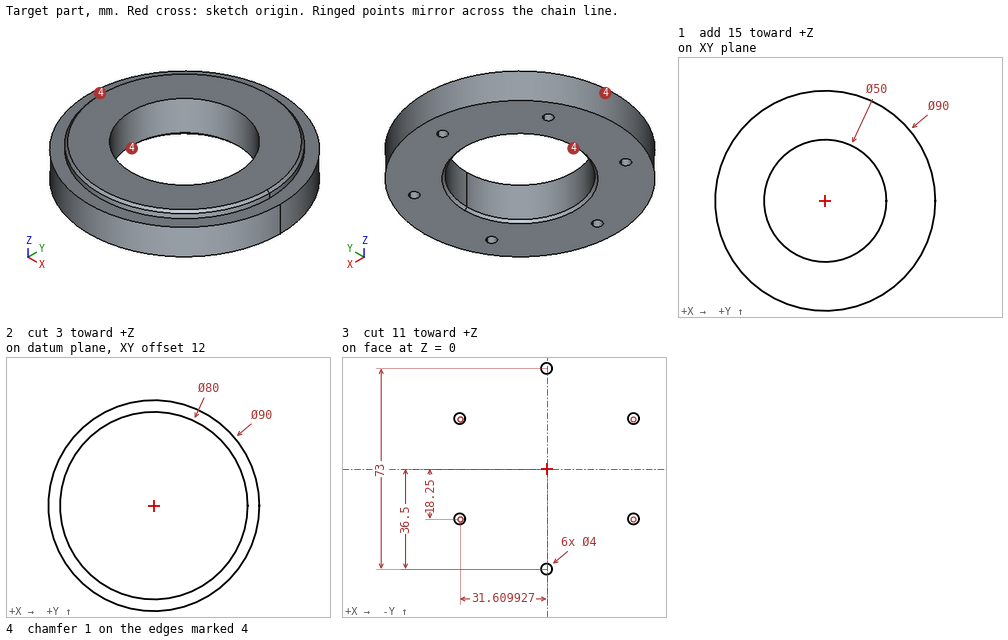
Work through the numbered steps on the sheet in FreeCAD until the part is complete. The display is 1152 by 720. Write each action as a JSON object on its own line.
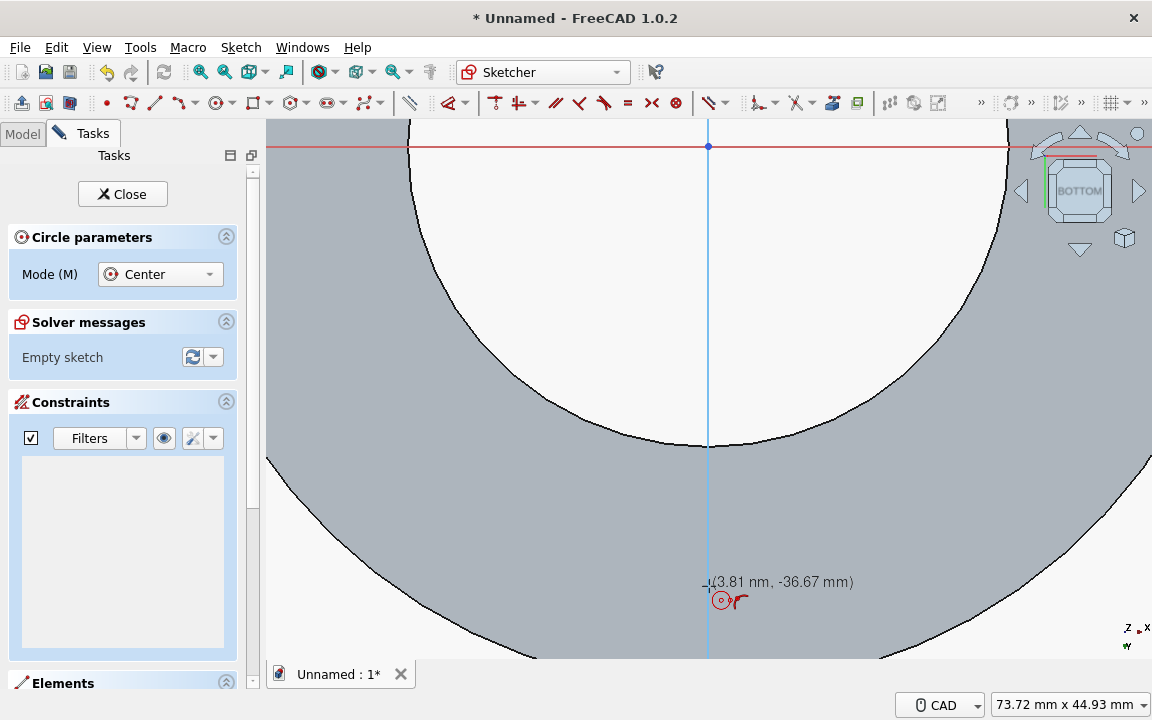
{"action": "left_click", "coordinate": [708, 585]}
{"action": "left_click", "coordinate": [725, 568]}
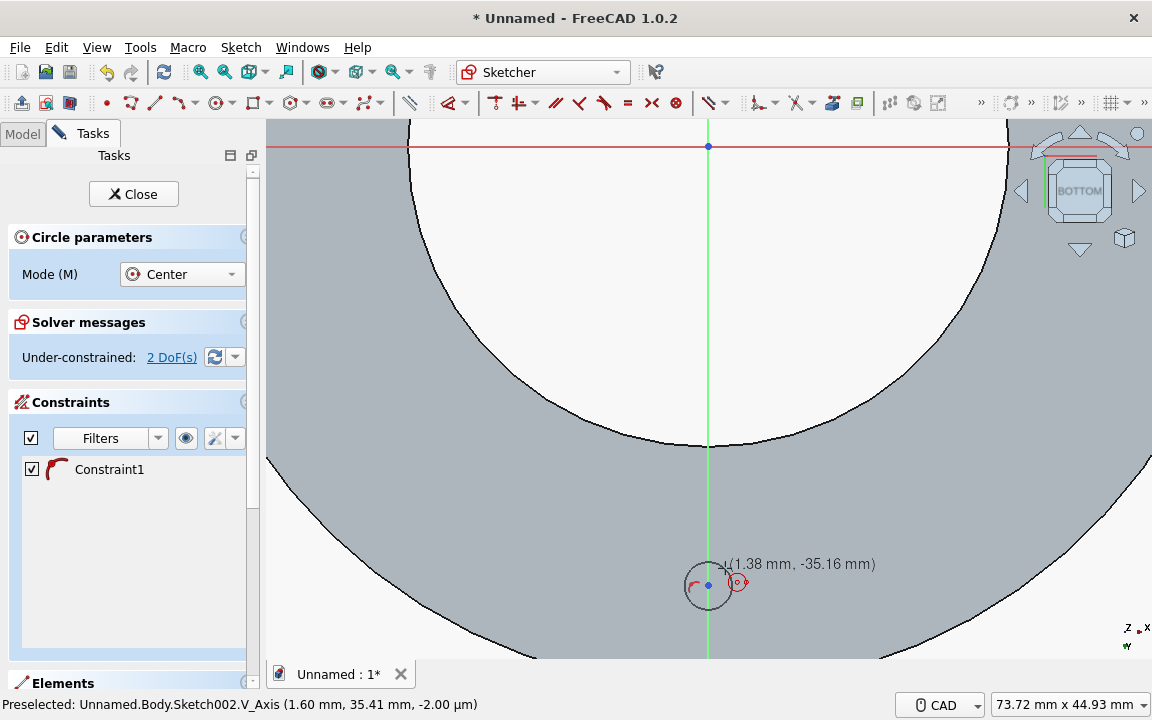
{"action": "left_click", "coordinate": [329, 366]}
{"action": "left_click", "coordinate": [345, 349]}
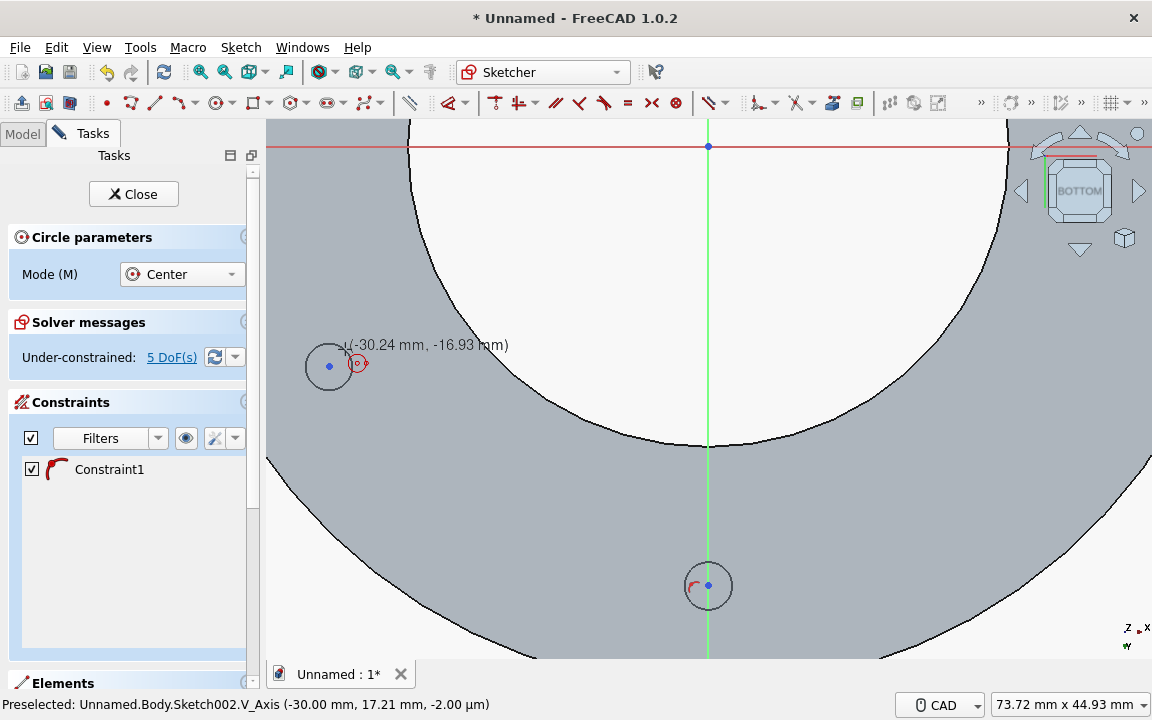
{"action": "scroll", "coordinate": [601, 530], "scroll_direction": "down", "scroll_amount": 5}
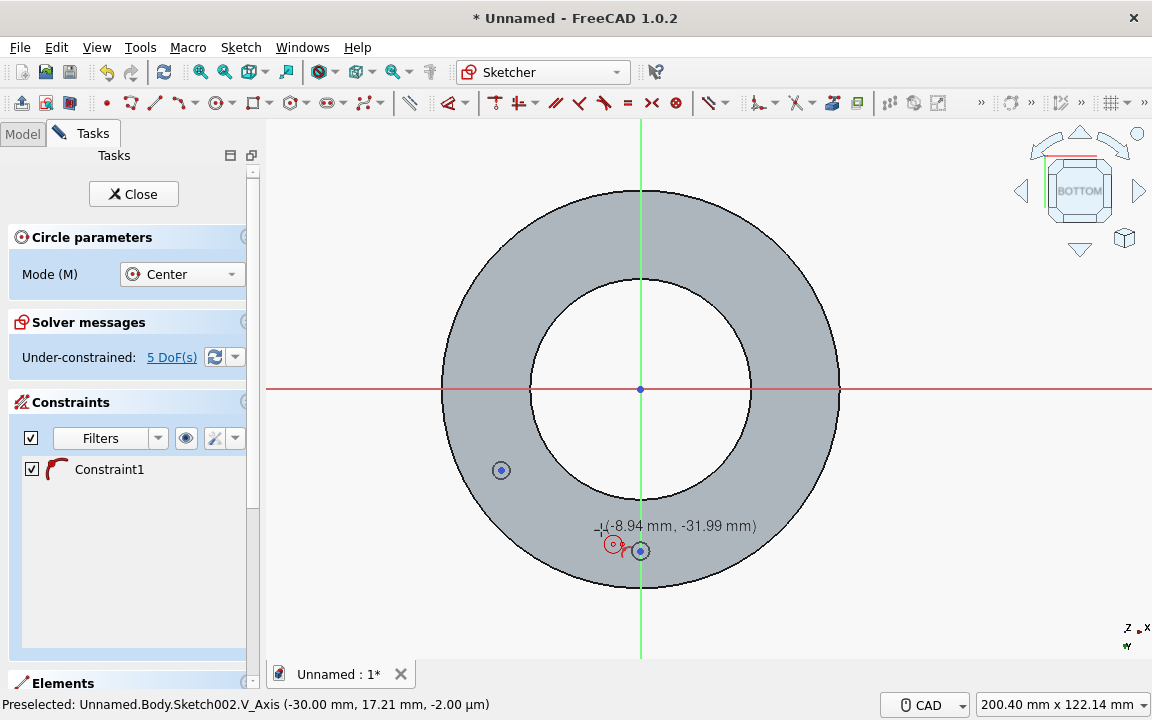
{"action": "scroll", "coordinate": [501, 309], "scroll_direction": "up", "scroll_amount": 5}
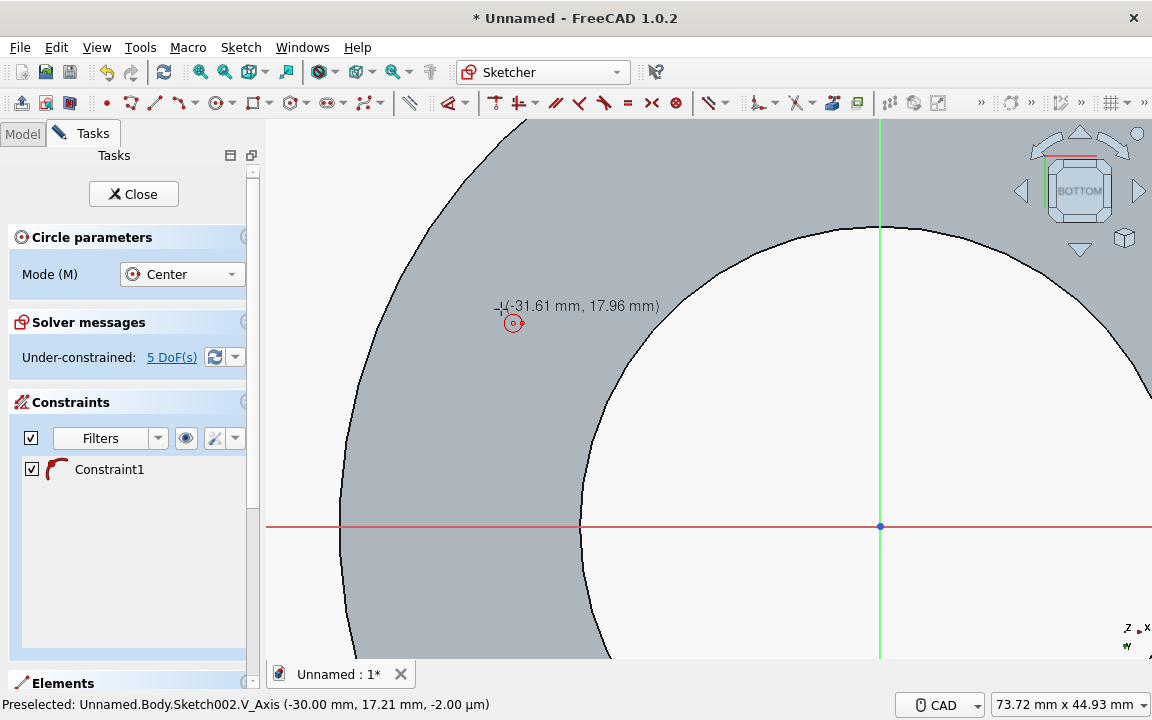
{"action": "left_click", "coordinate": [501, 308]}
{"action": "left_click", "coordinate": [518, 291]}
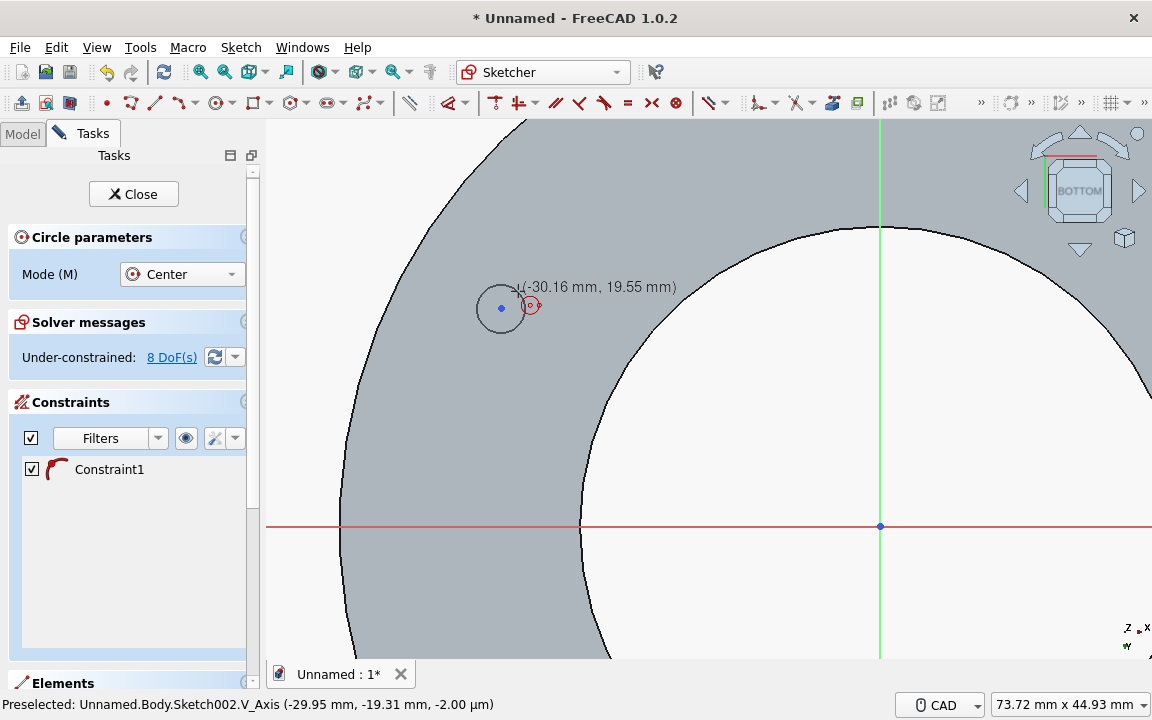
{"action": "scroll", "coordinate": [501, 309], "scroll_direction": "down", "scroll_amount": 5}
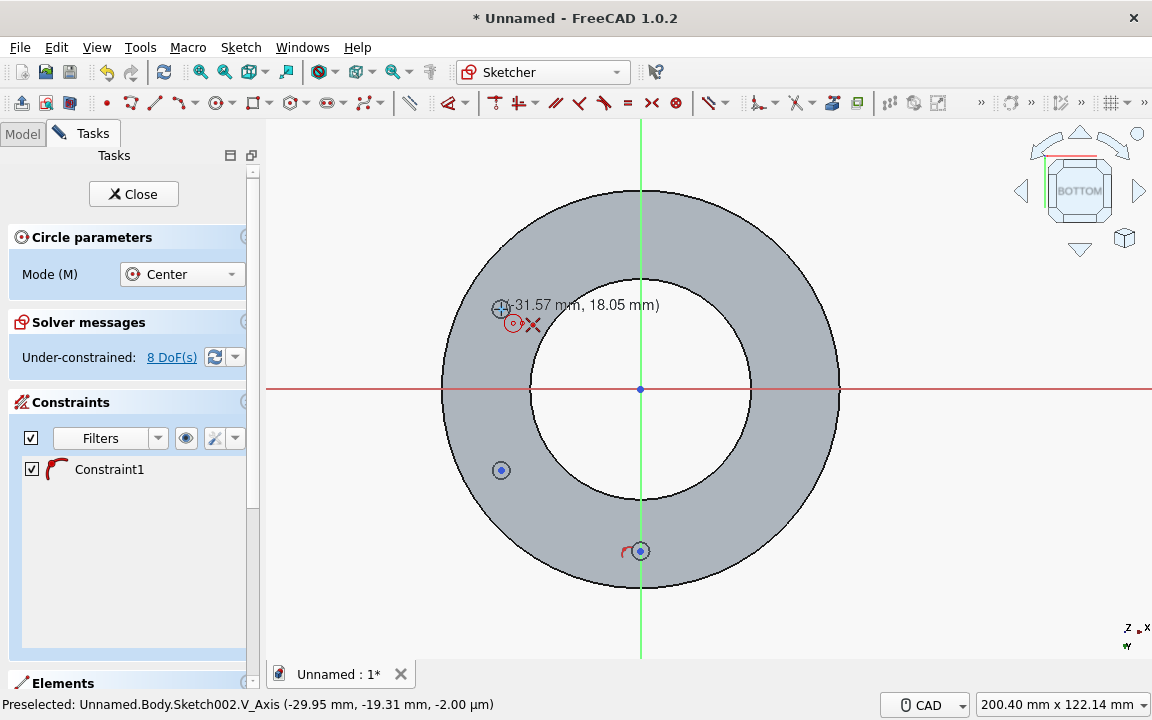
{"action": "scroll", "coordinate": [641, 228], "scroll_direction": "up", "scroll_amount": 5}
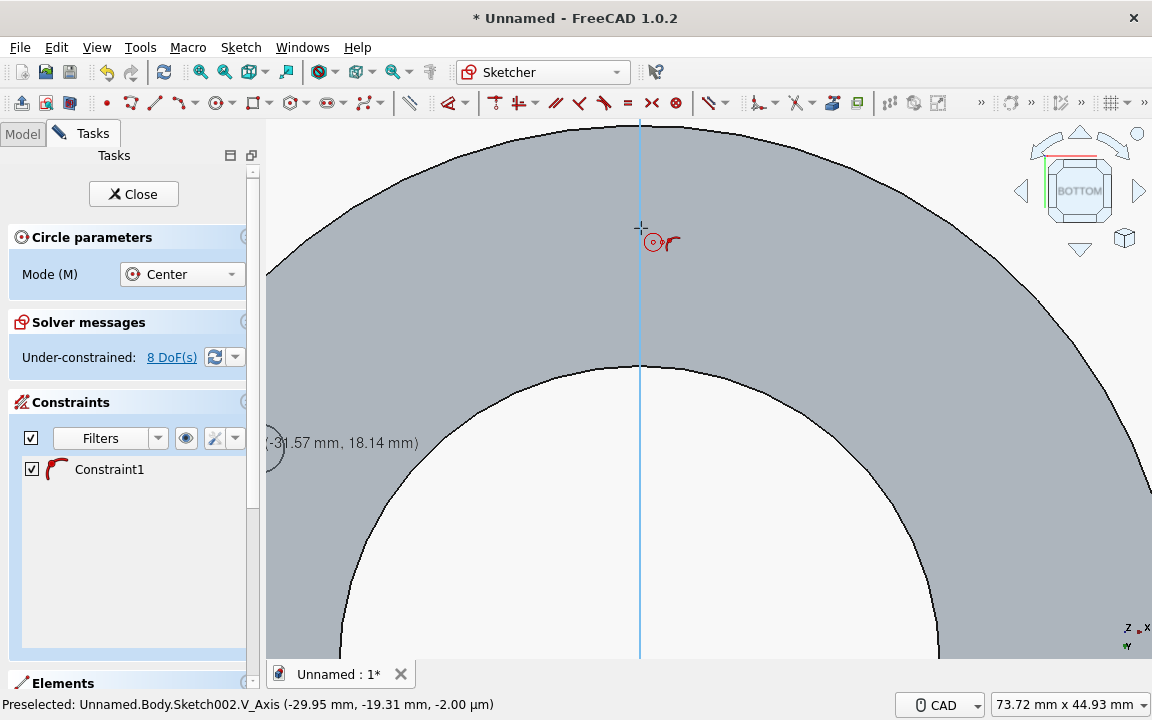
{"action": "left_click", "coordinate": [640, 228]}
{"action": "left_click", "coordinate": [657, 211]}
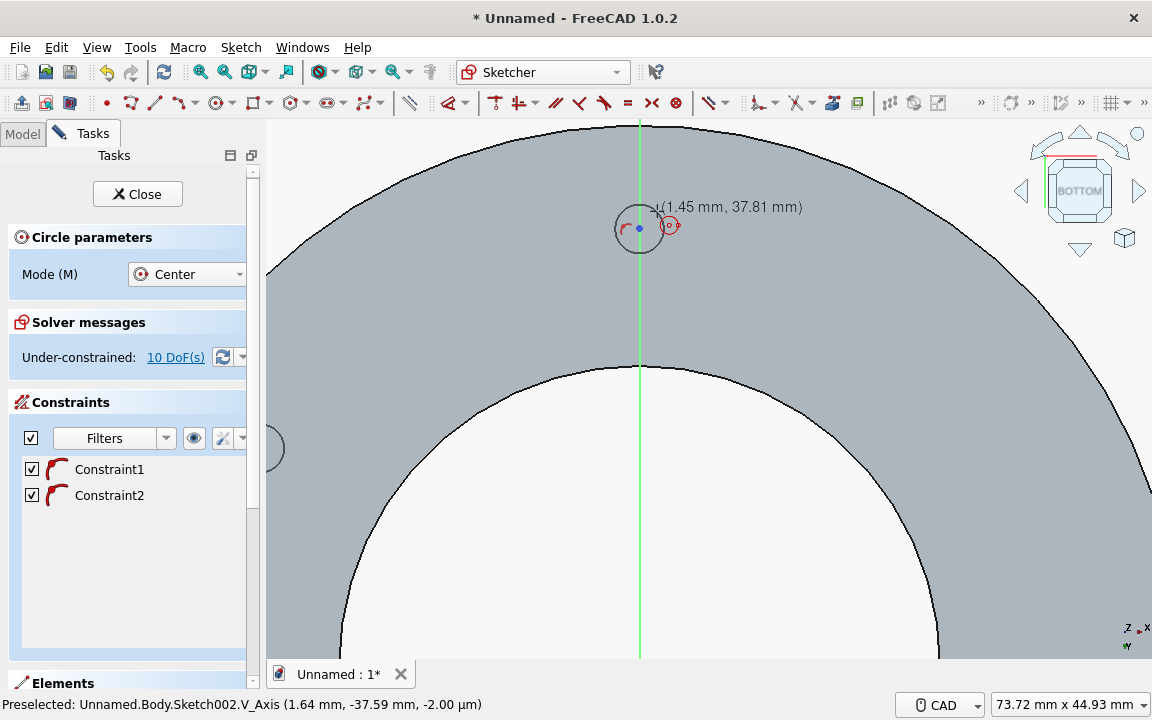
{"action": "scroll", "coordinate": [641, 228], "scroll_direction": "down", "scroll_amount": 5}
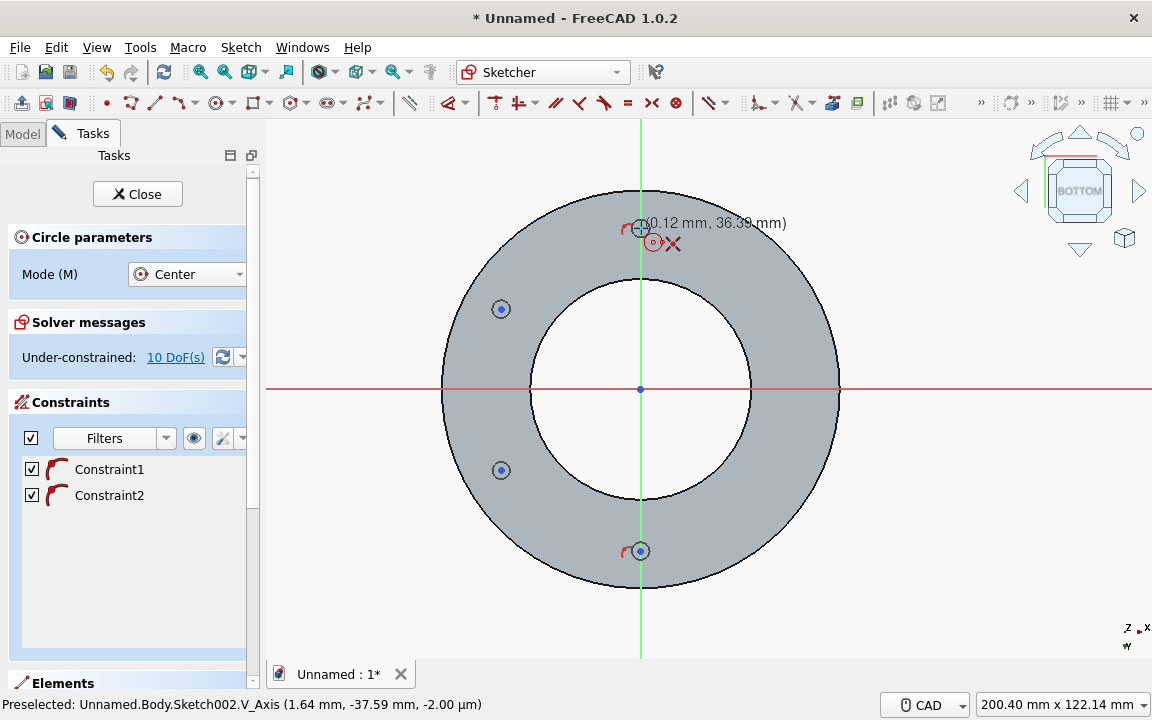
{"action": "scroll", "coordinate": [780, 309], "scroll_direction": "up", "scroll_amount": 5}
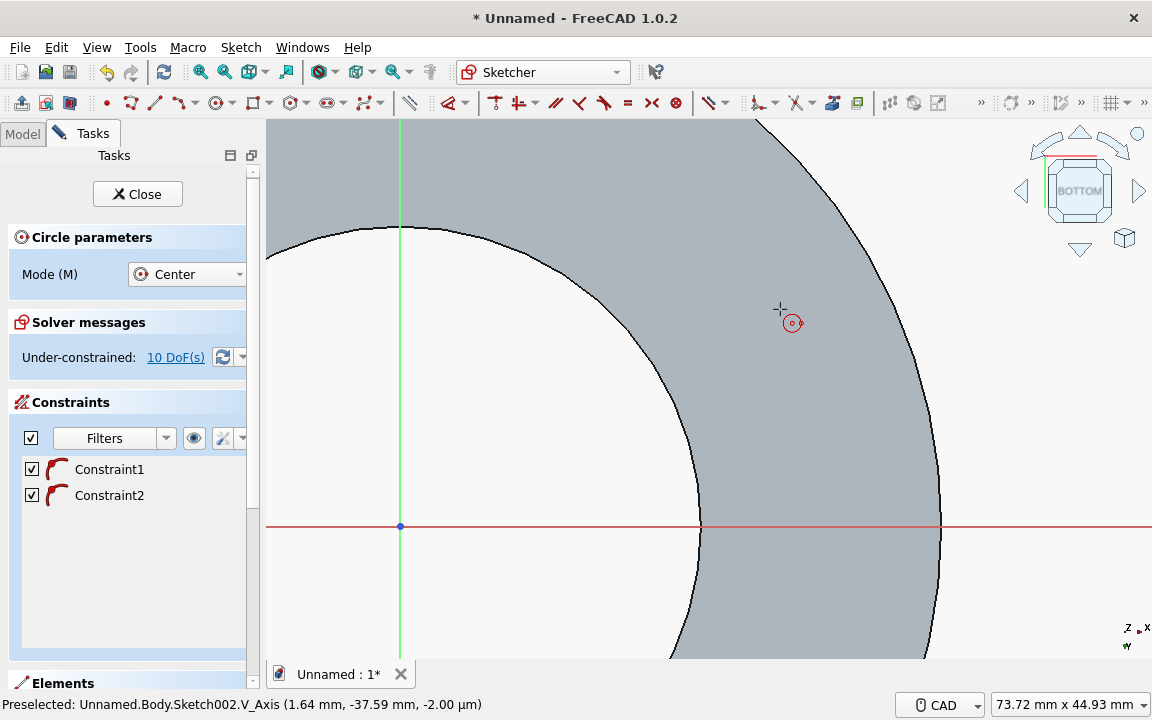
{"action": "left_click", "coordinate": [780, 308]}
{"action": "left_click", "coordinate": [797, 291]}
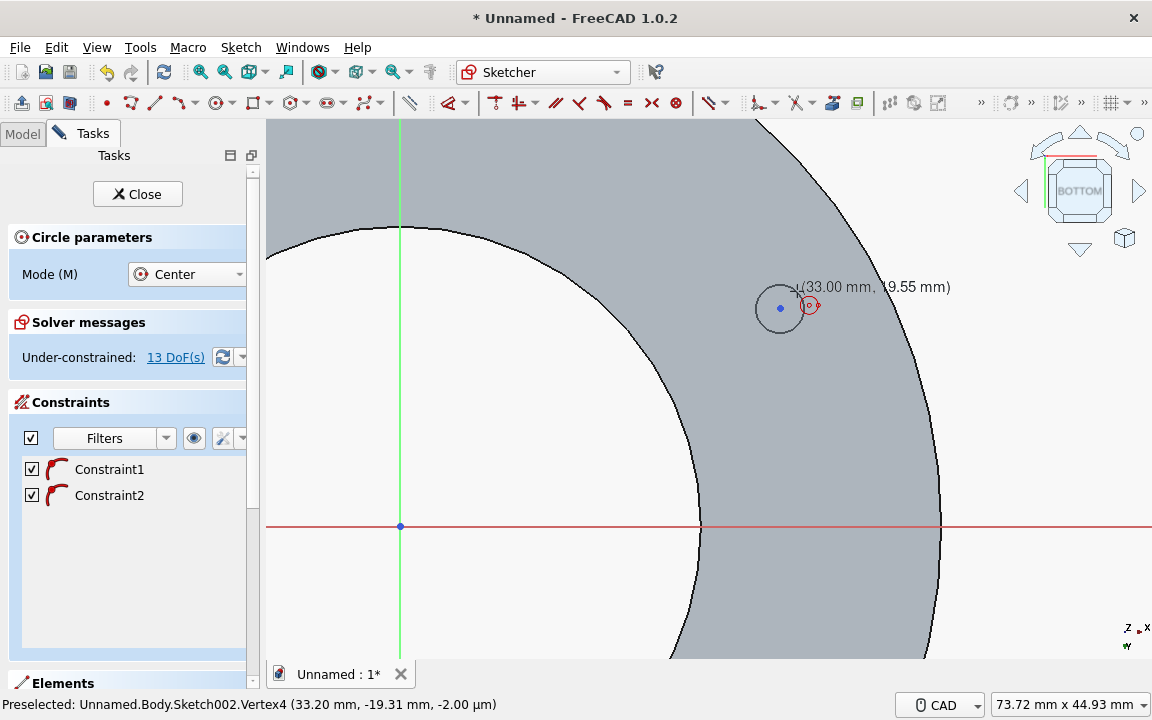
{"action": "scroll", "coordinate": [780, 309], "scroll_direction": "down", "scroll_amount": 5}